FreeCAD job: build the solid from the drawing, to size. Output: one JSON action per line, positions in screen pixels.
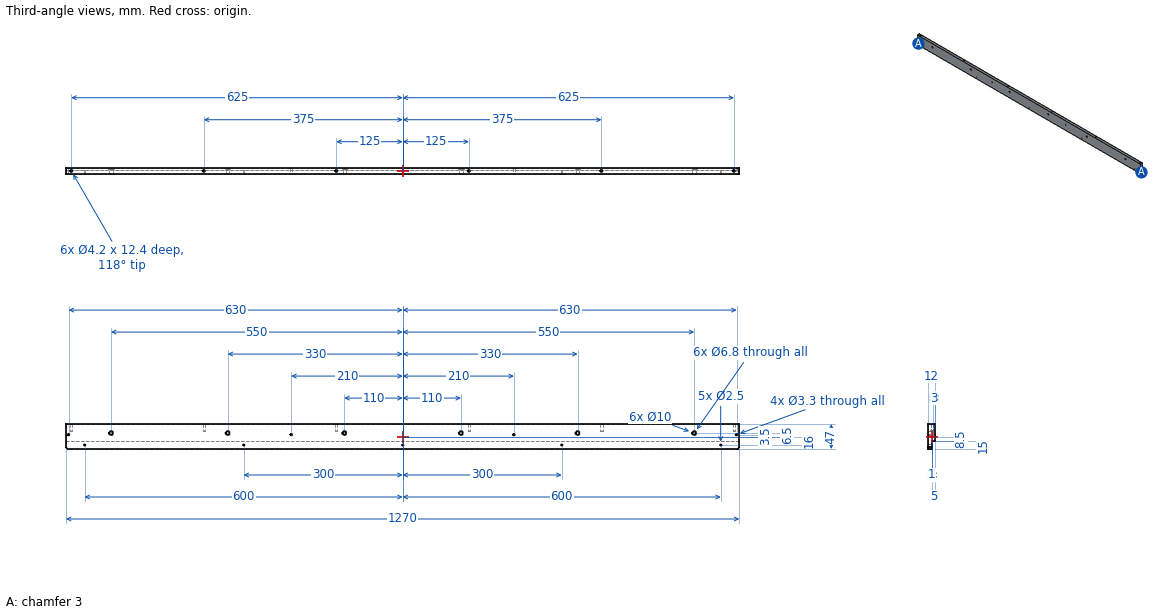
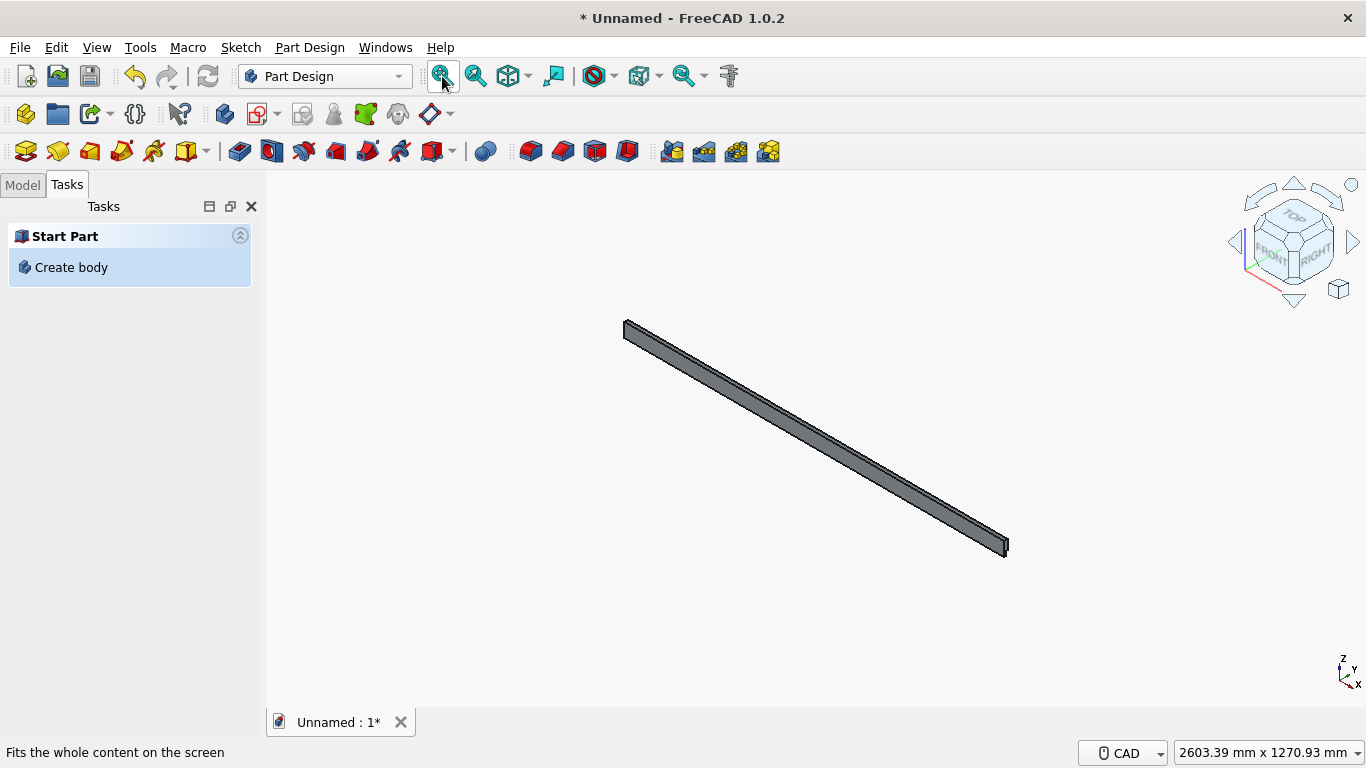
{"action": "scroll", "coordinate": [626, 337], "scroll_direction": "up", "scroll_amount": 14}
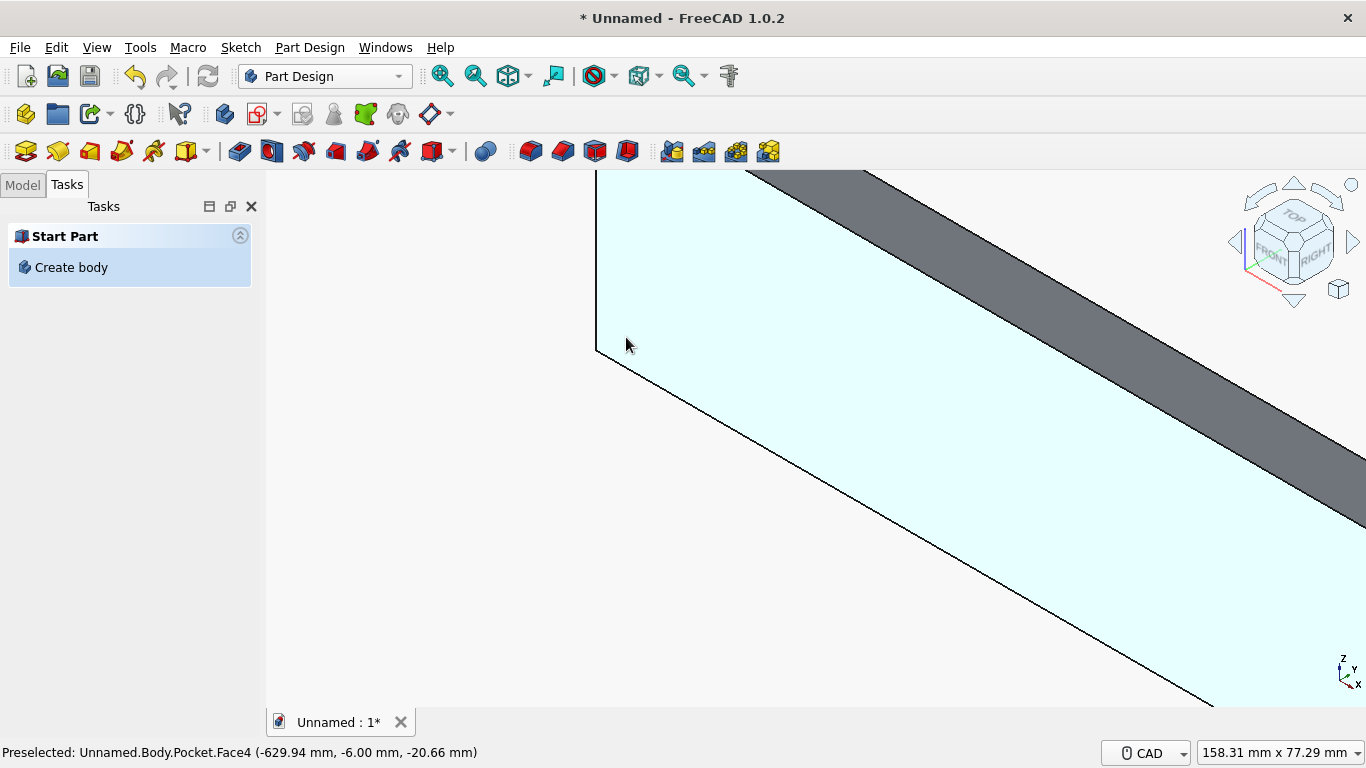
{"action": "key", "text": "v f"}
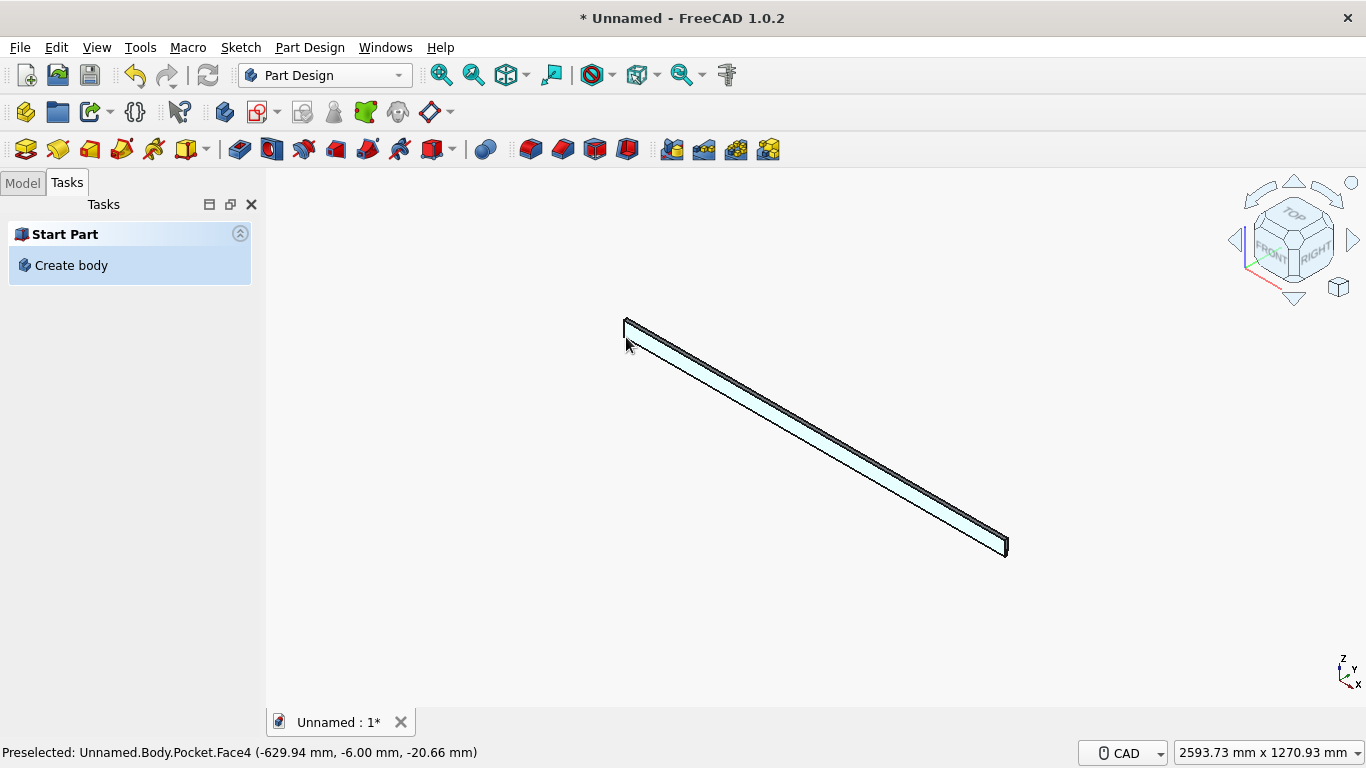
{"action": "key", "text": "2"}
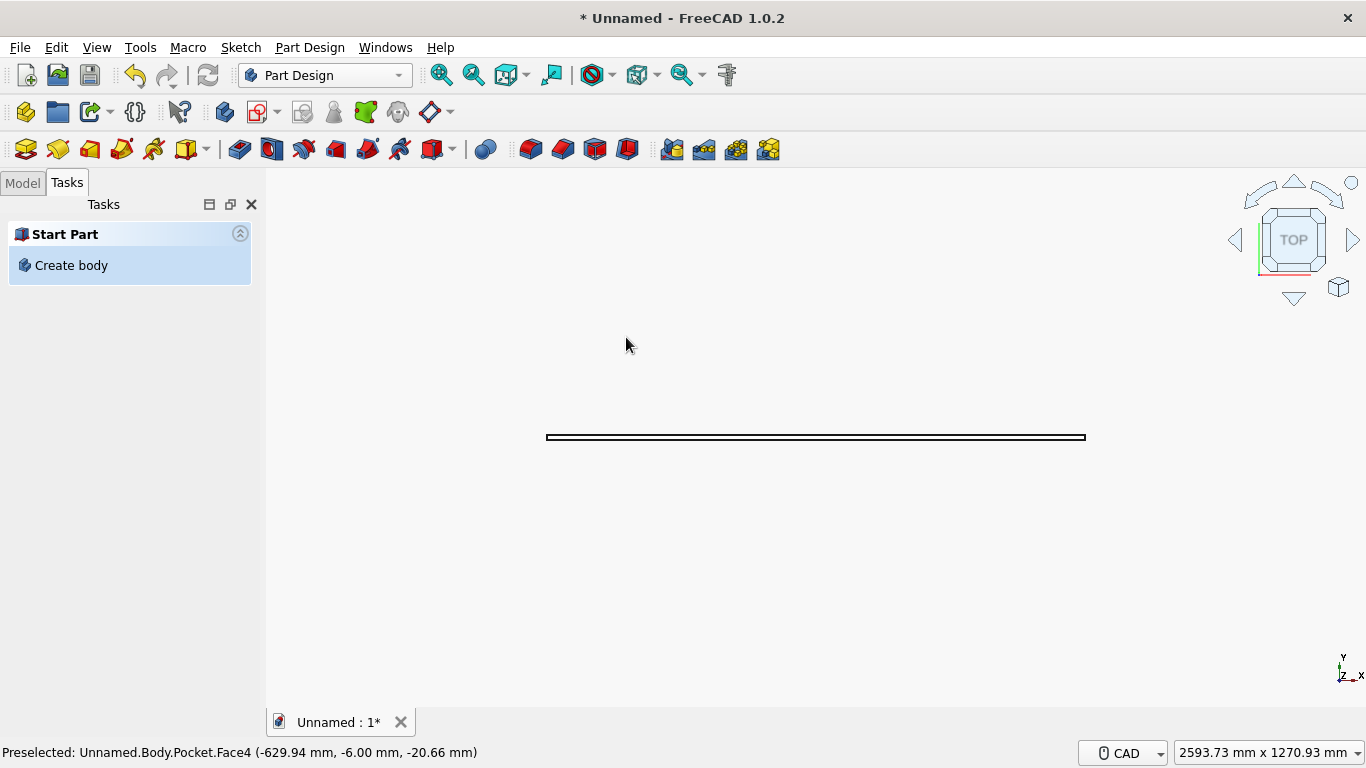
{"action": "scroll", "coordinate": [547, 438], "scroll_direction": "up", "scroll_amount": 14}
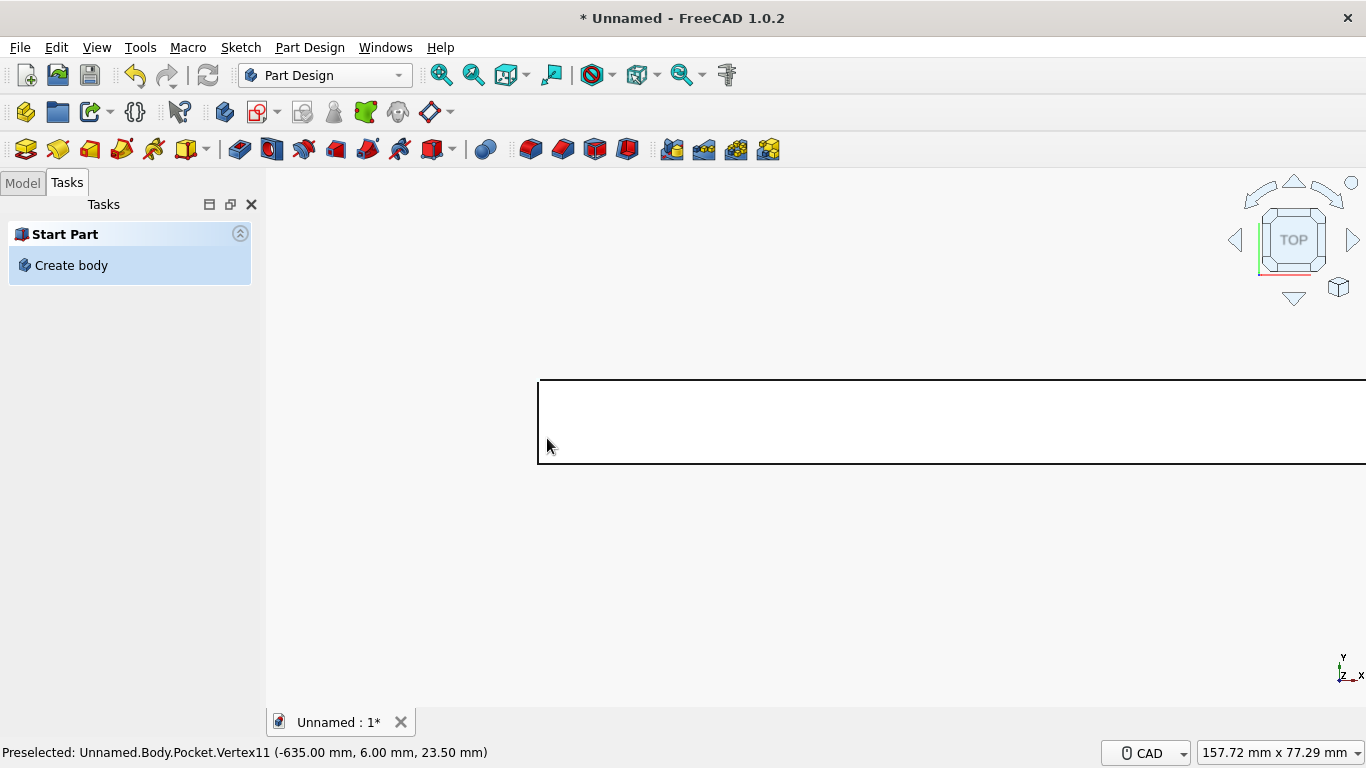
{"action": "left_click", "coordinate": [442, 76]}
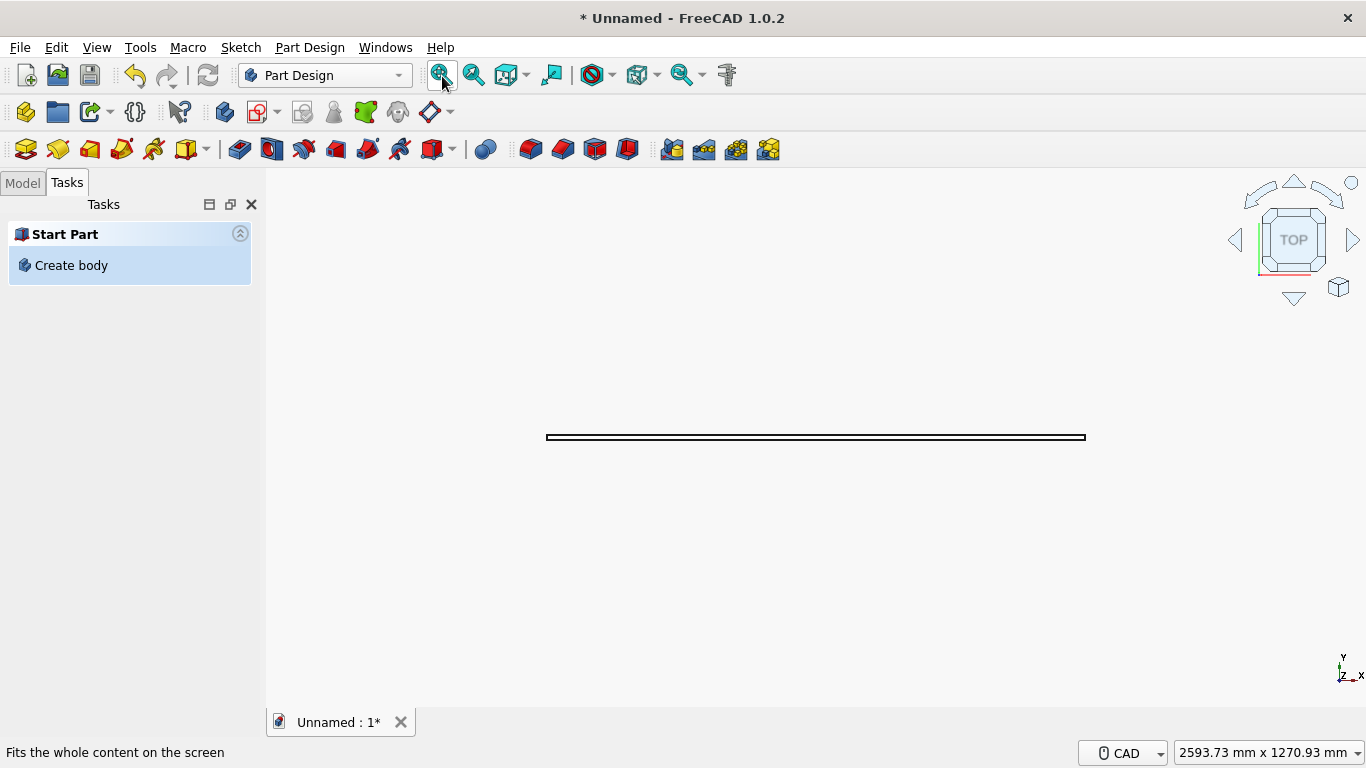
{"action": "key", "text": "1"}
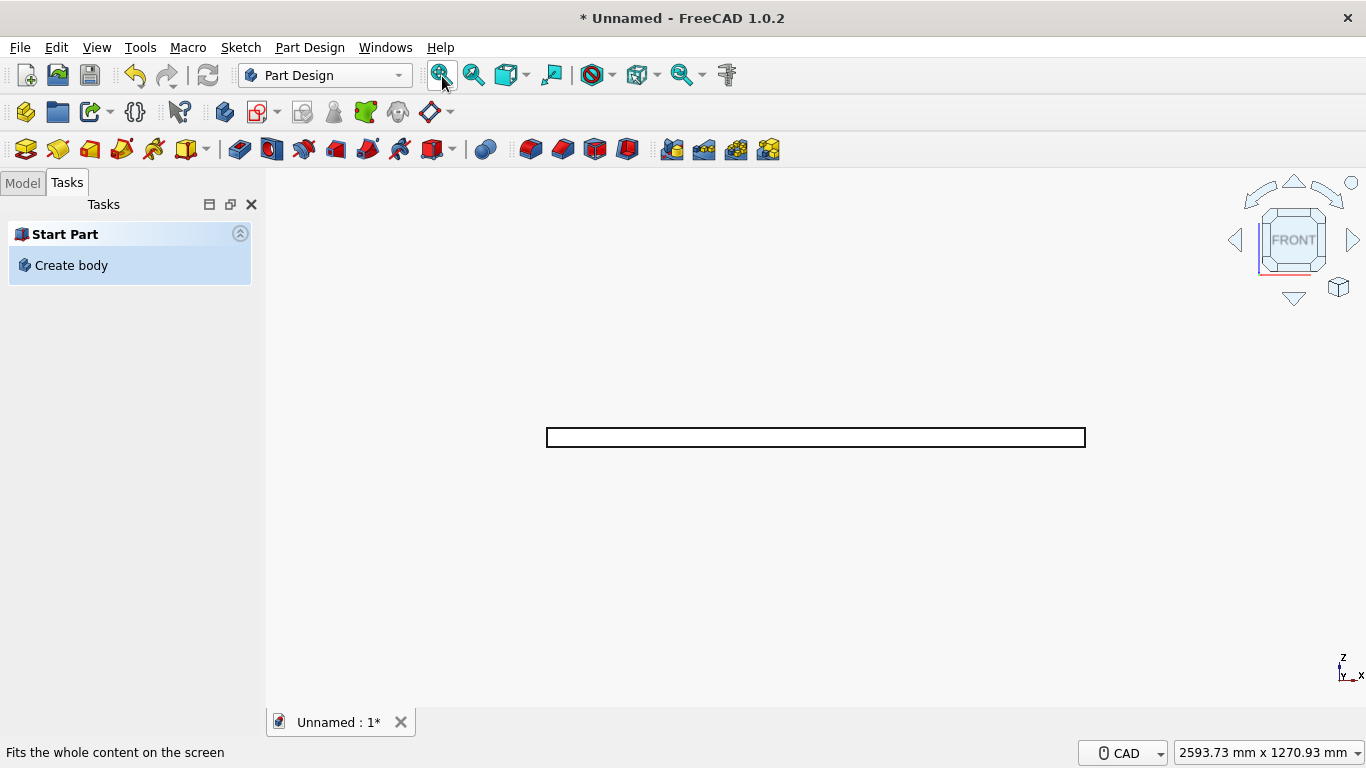
{"action": "scroll", "coordinate": [547, 446], "scroll_direction": "up", "scroll_amount": 14}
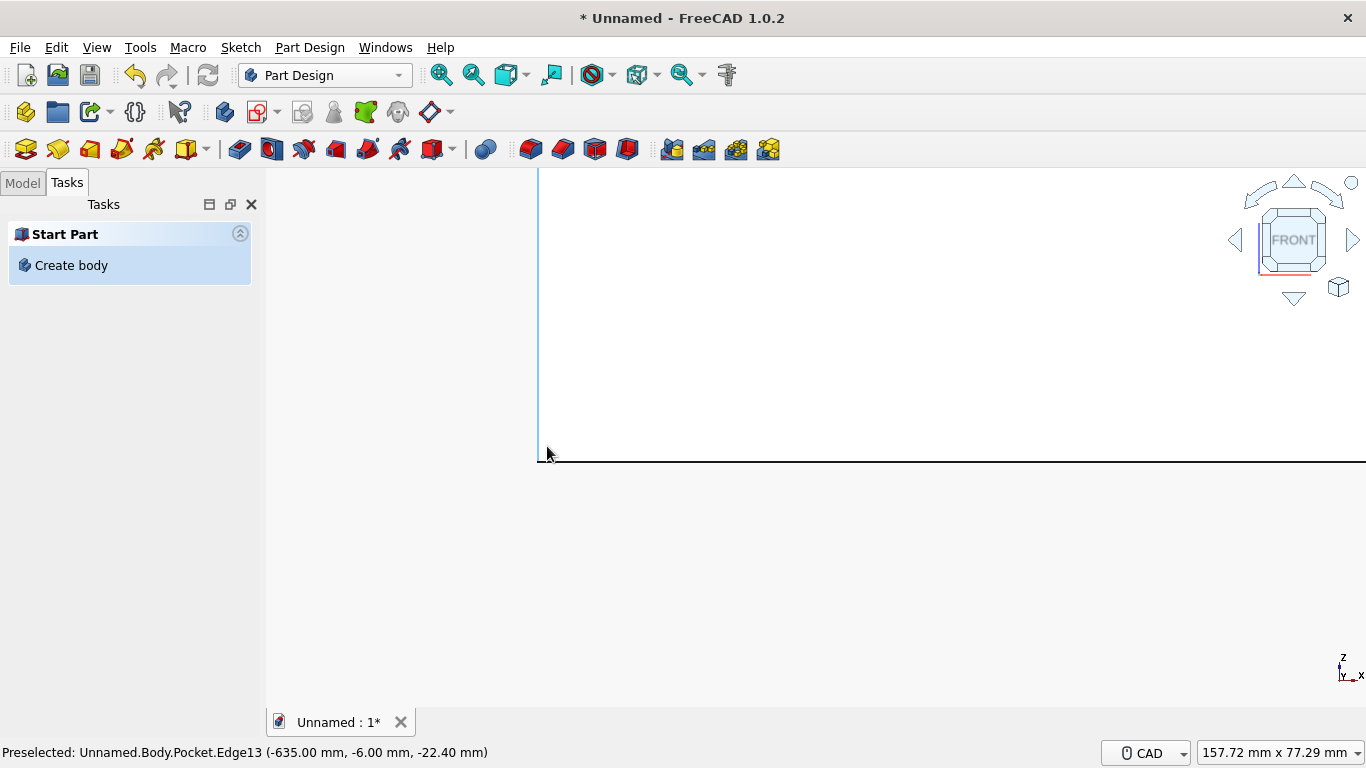
{"action": "left_click", "coordinate": [442, 76]}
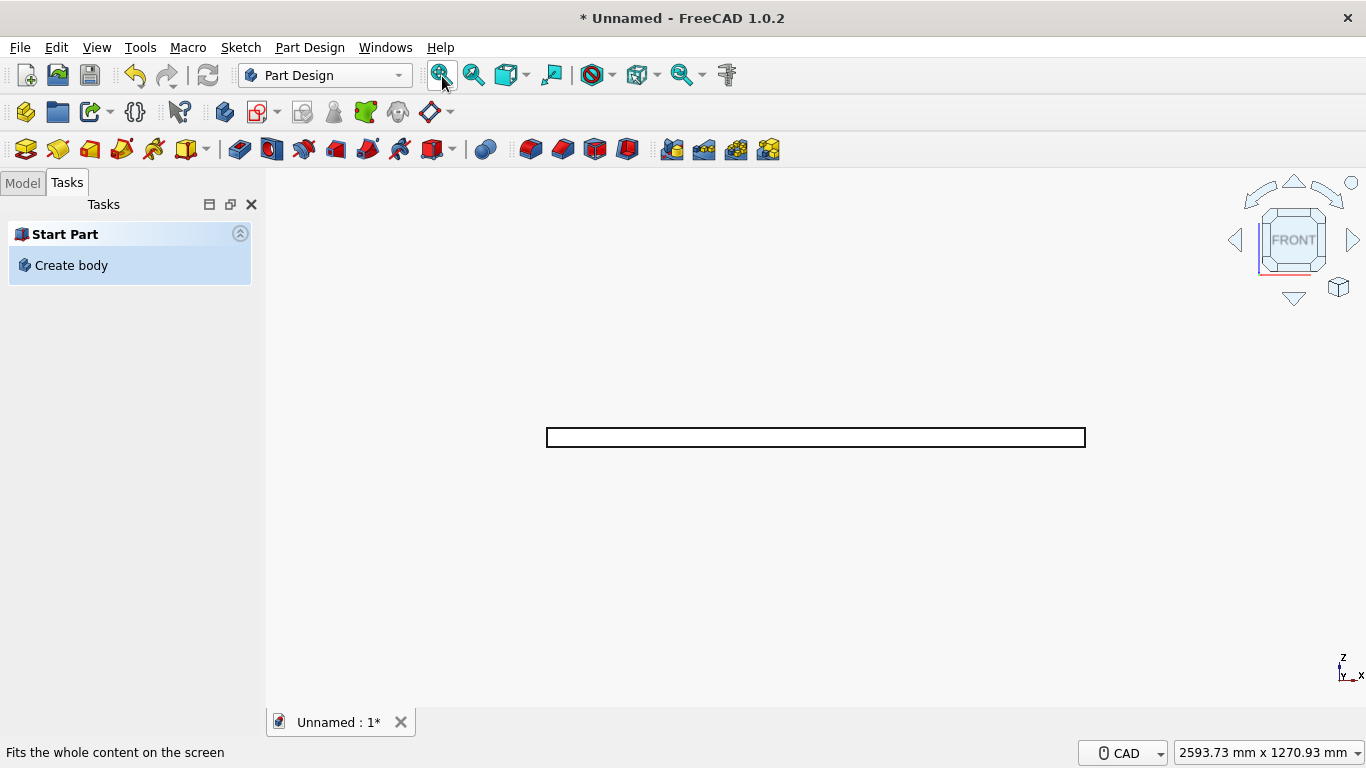
{"action": "key", "text": "3"}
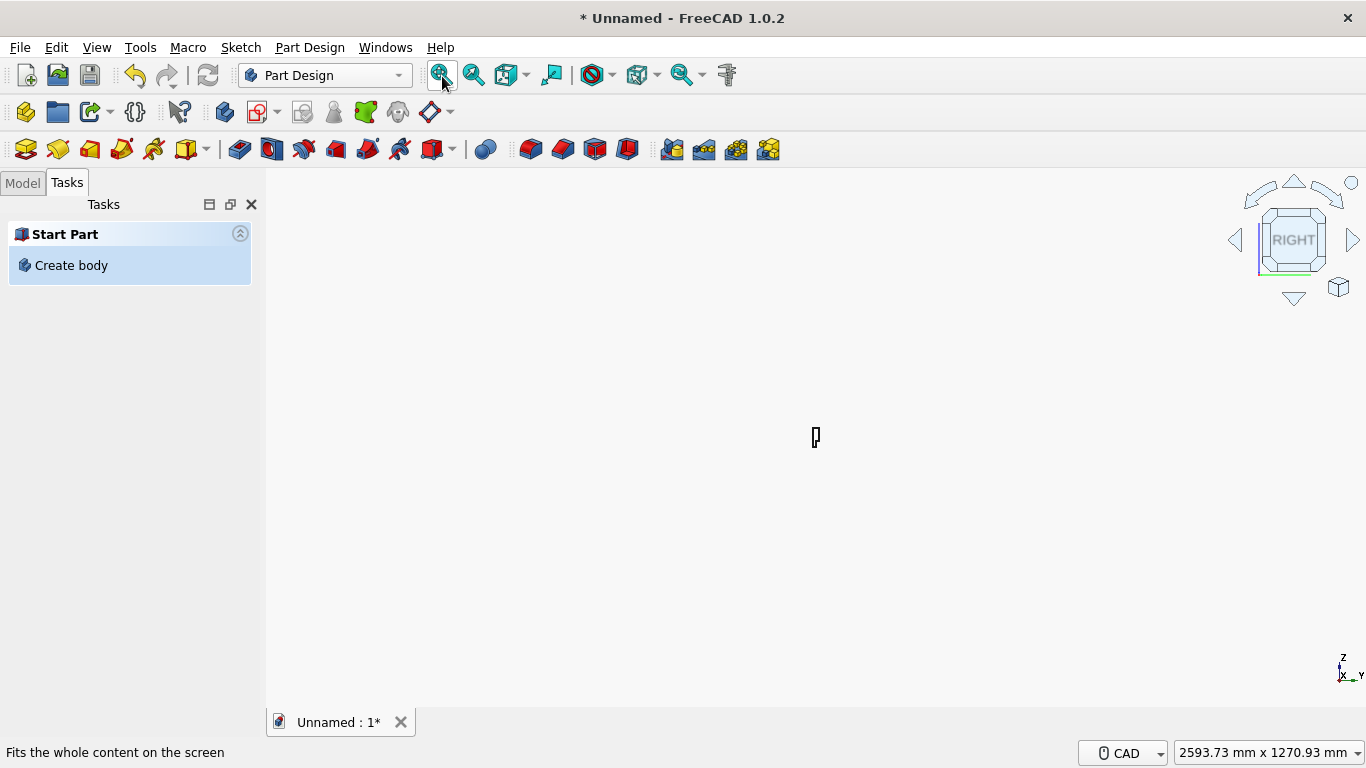
{"action": "left_click", "coordinate": [442, 76]}